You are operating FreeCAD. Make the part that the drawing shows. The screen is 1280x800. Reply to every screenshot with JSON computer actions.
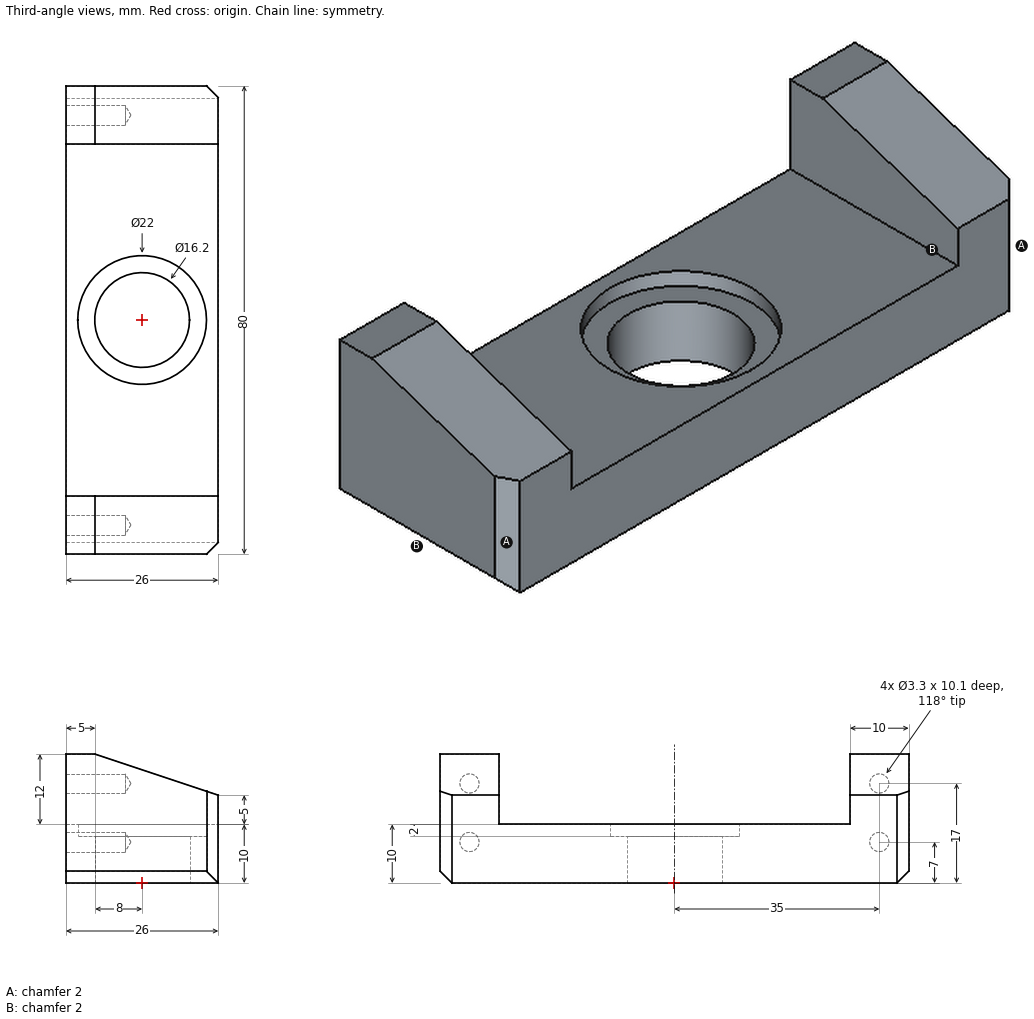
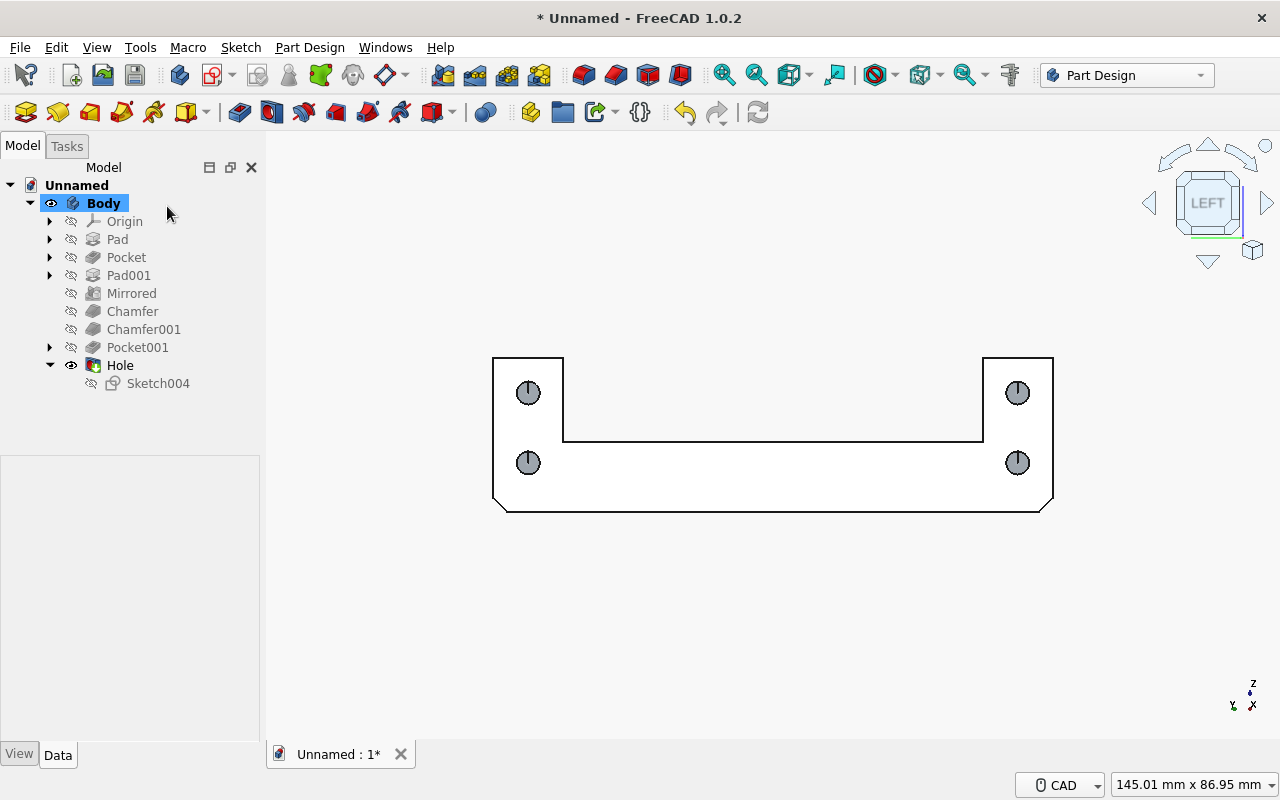
{"action": "key", "text": "0"}